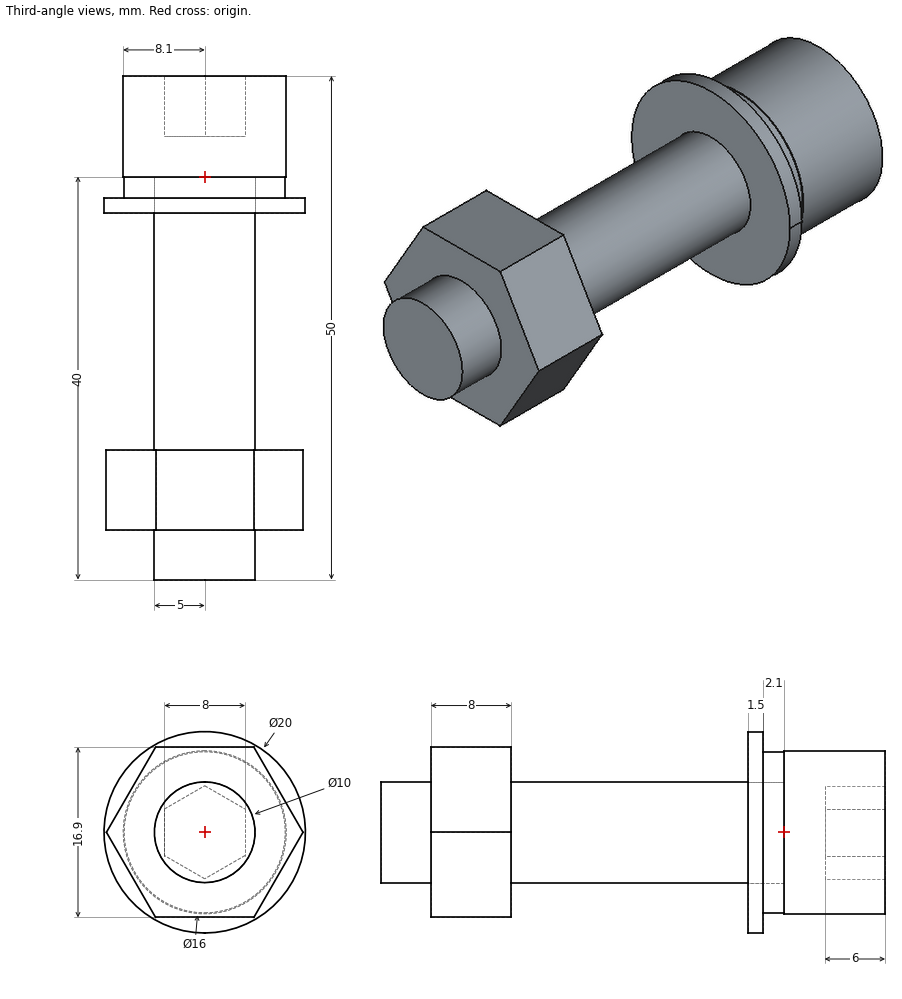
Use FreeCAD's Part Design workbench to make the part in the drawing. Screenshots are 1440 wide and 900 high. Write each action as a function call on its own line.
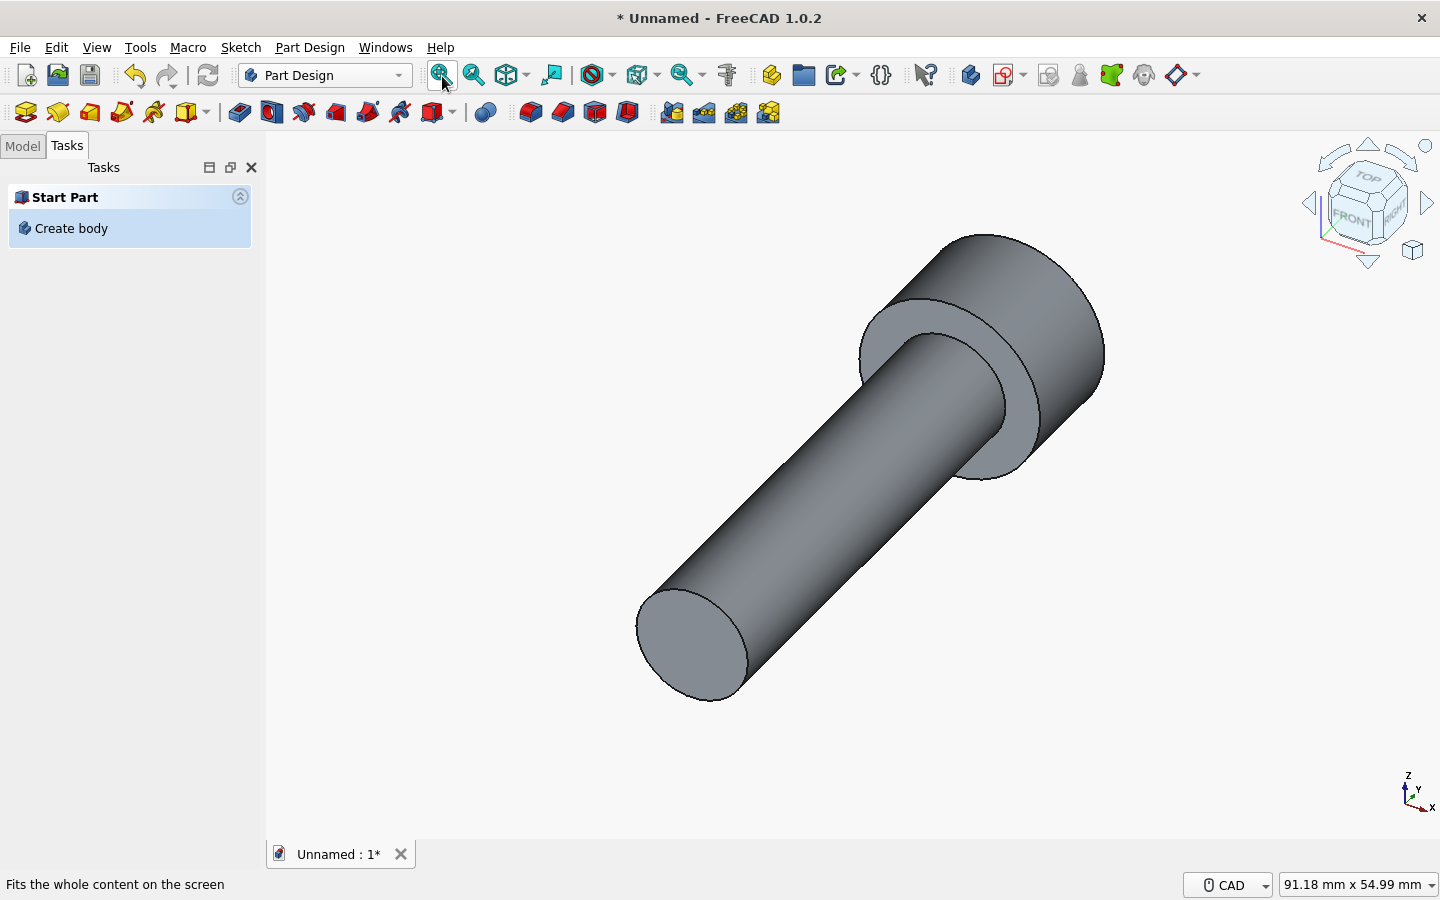
key(4)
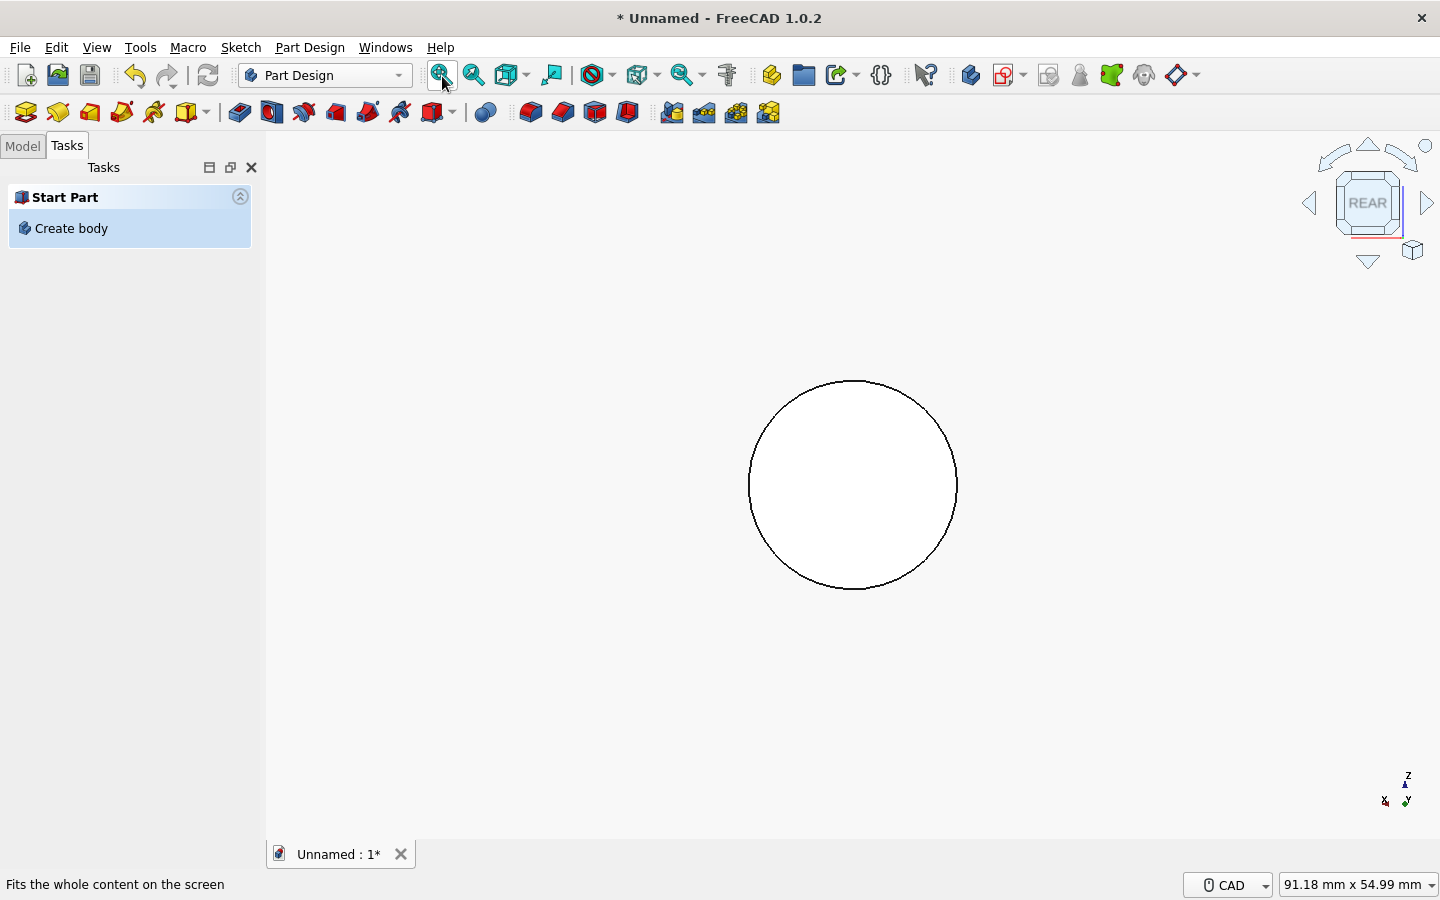
click(442, 76)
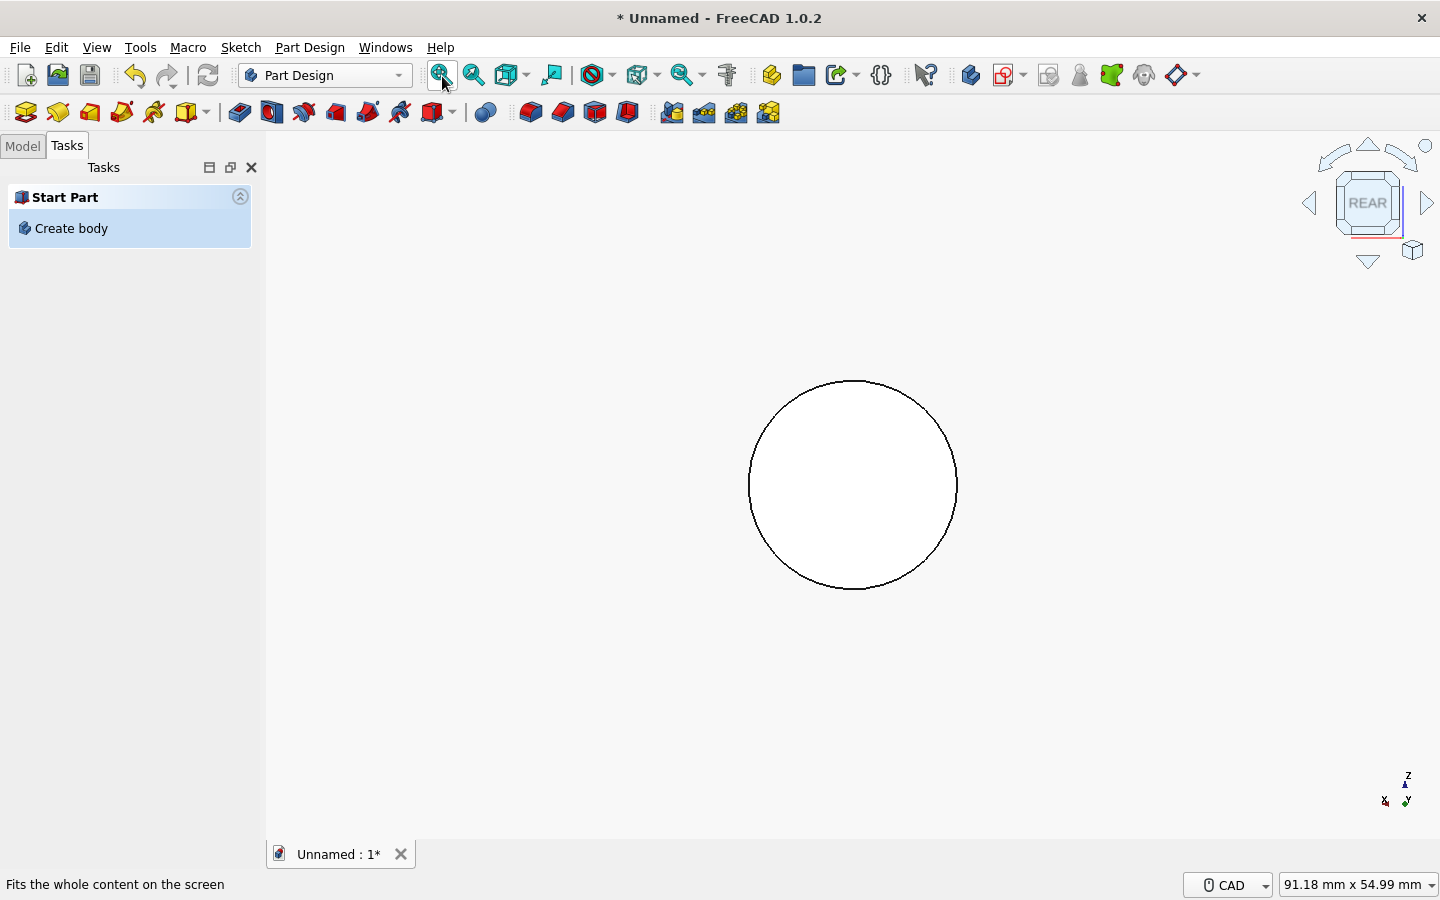
click(853, 484)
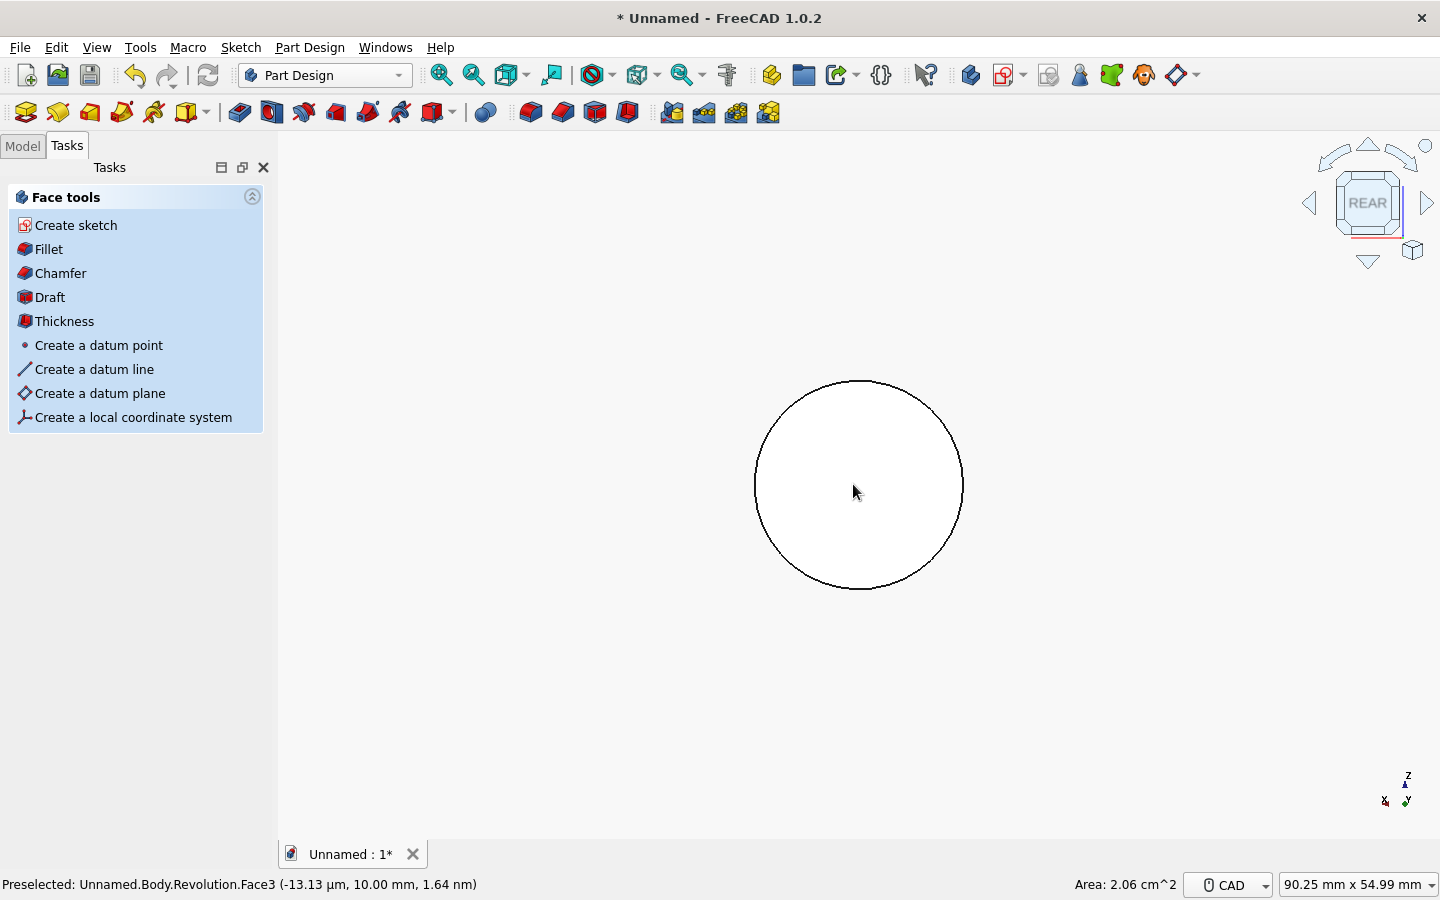
click(1004, 76)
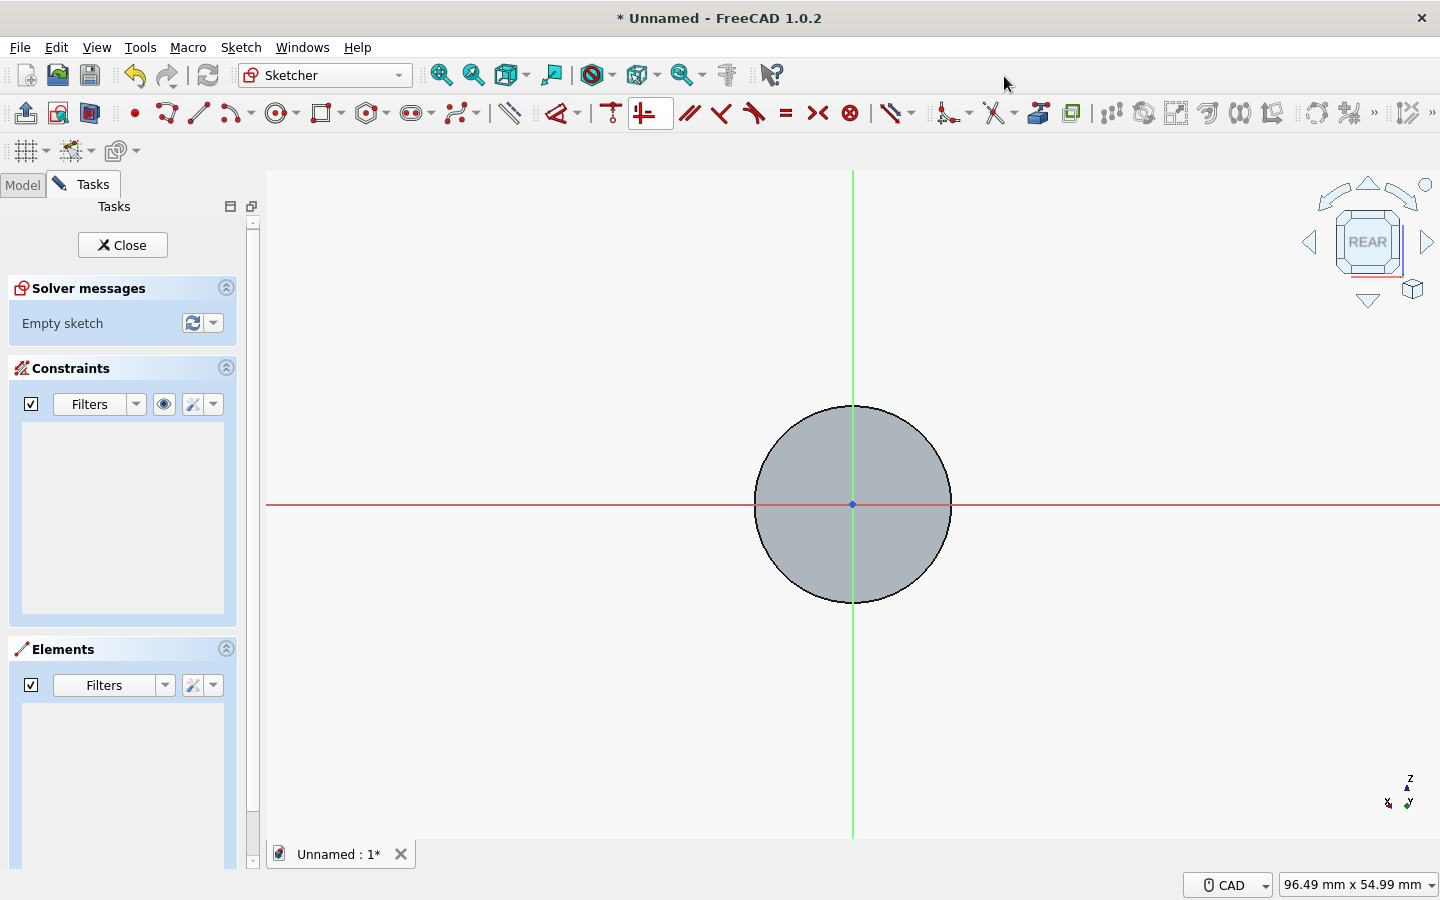
scroll(875, 505, up, 7)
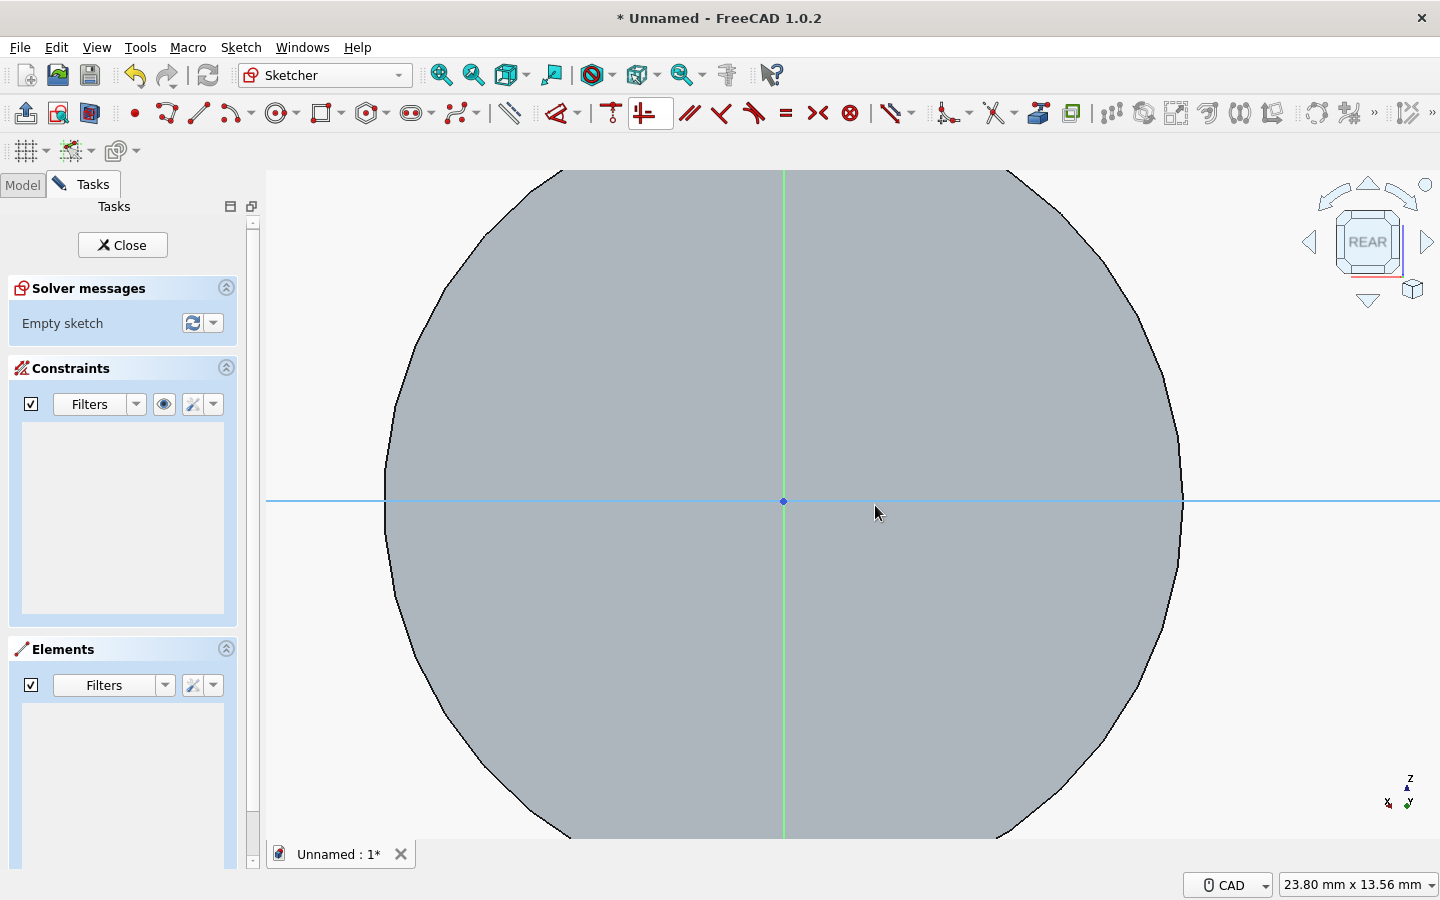
click(366, 114)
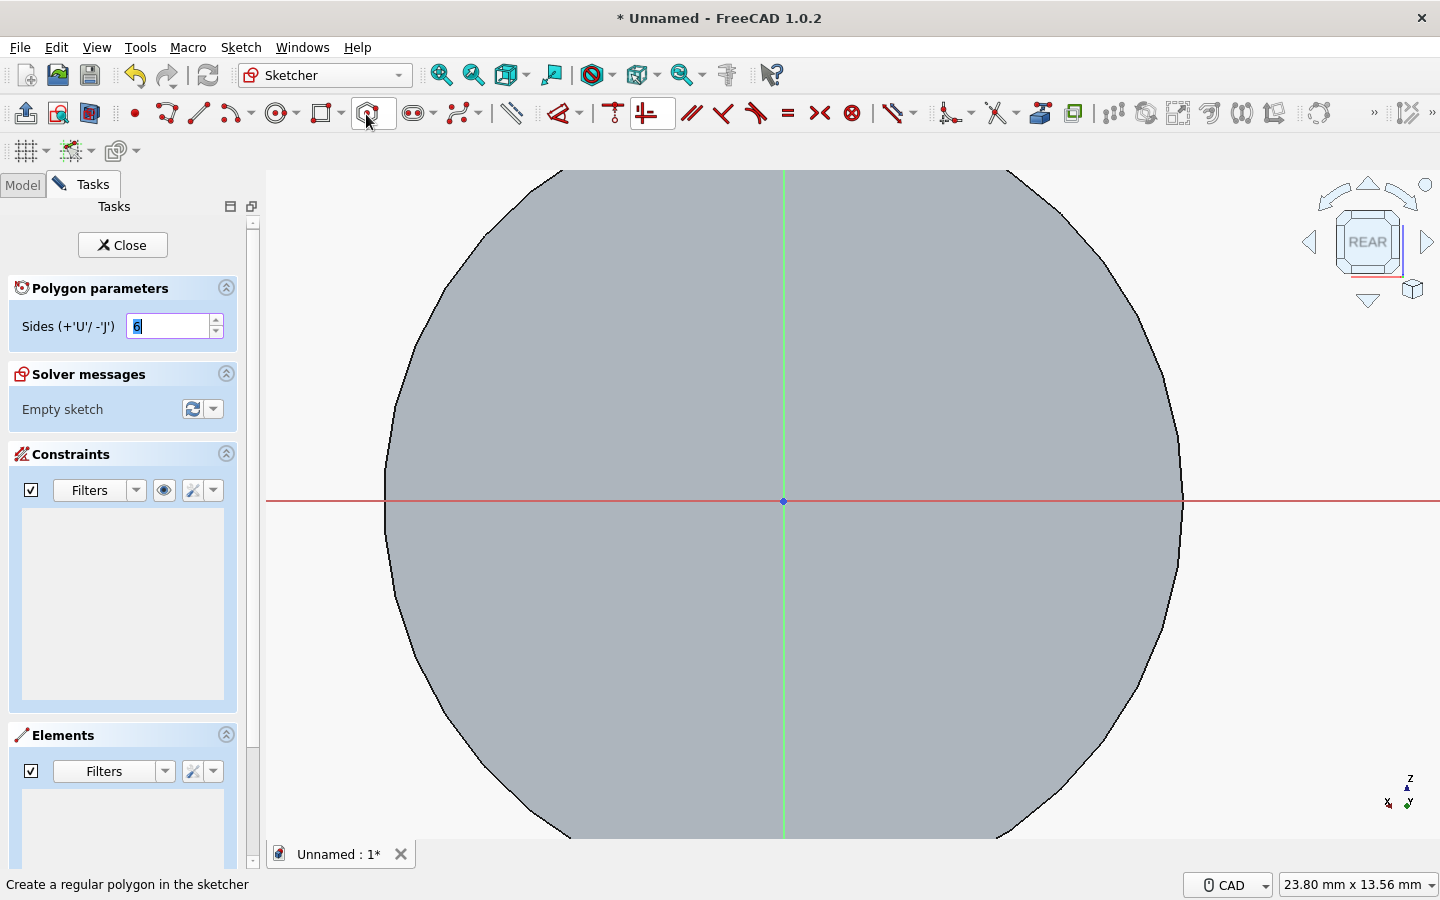
click(784, 501)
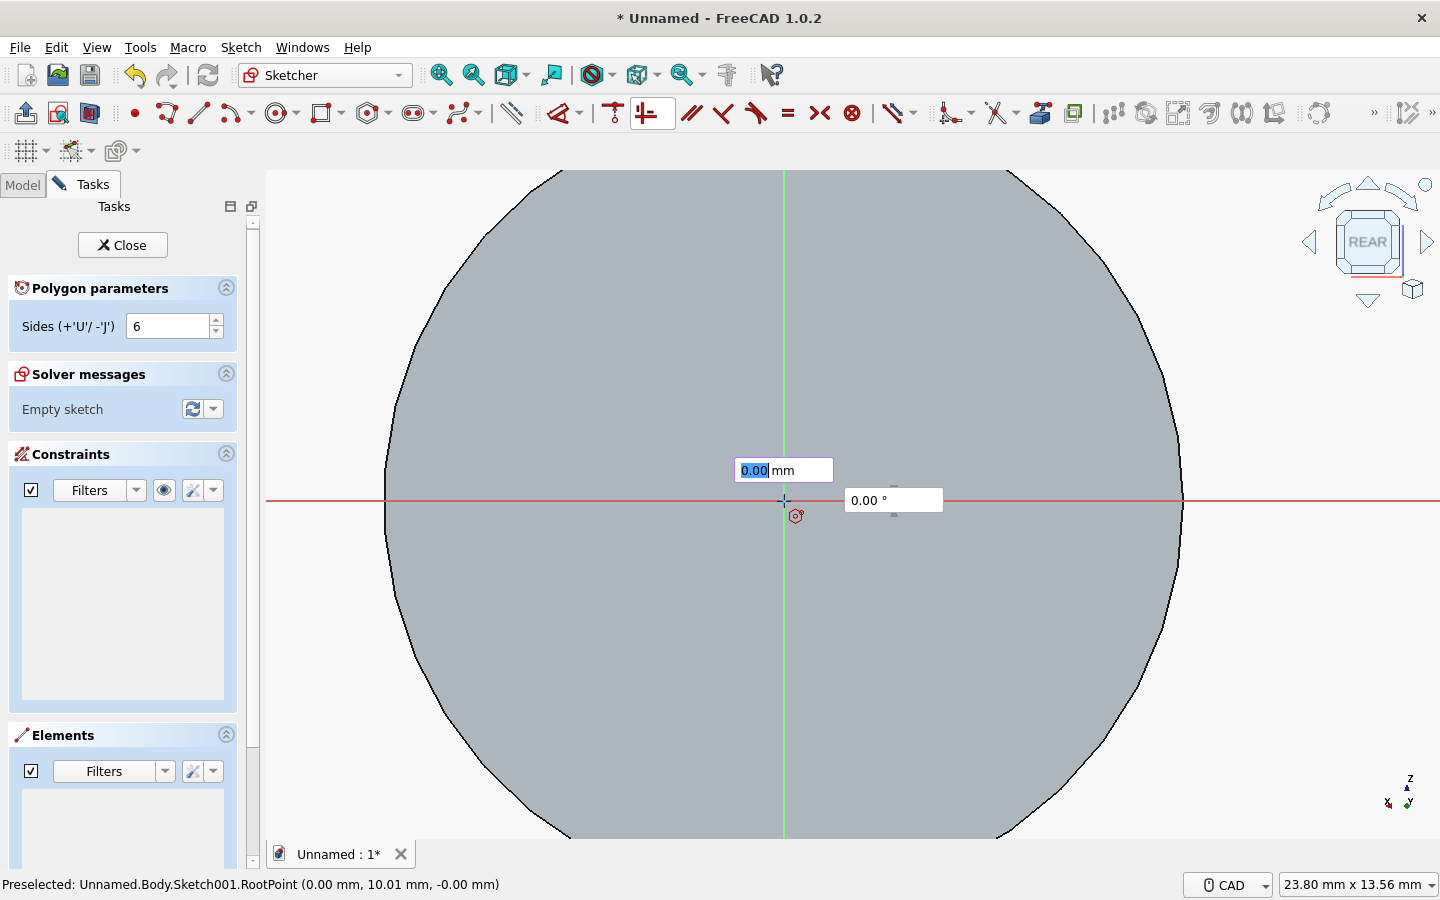
click(784, 729)
right_click(784, 729)